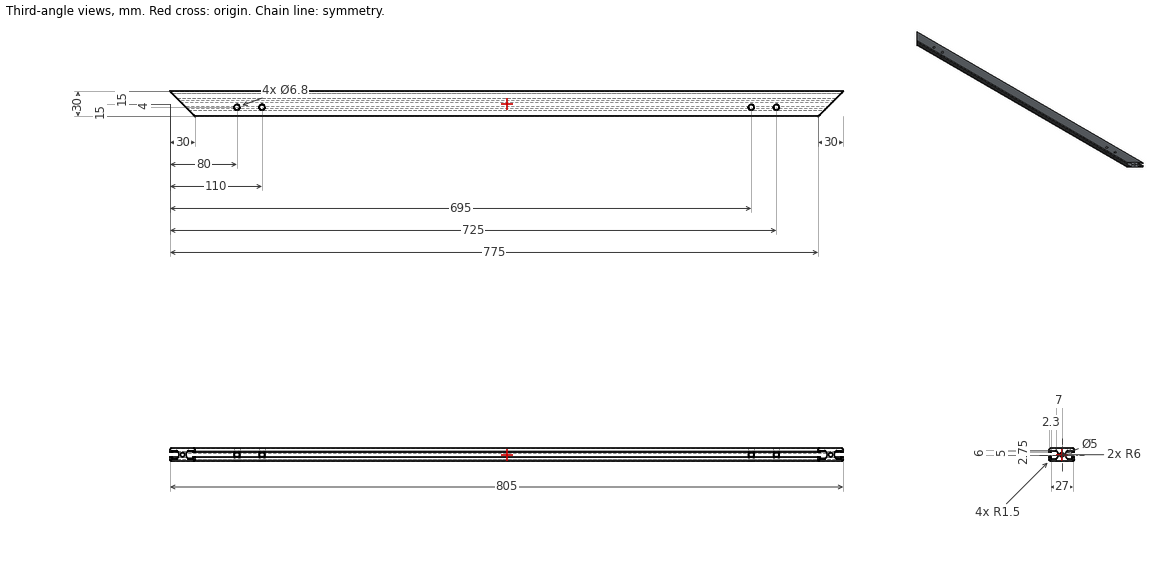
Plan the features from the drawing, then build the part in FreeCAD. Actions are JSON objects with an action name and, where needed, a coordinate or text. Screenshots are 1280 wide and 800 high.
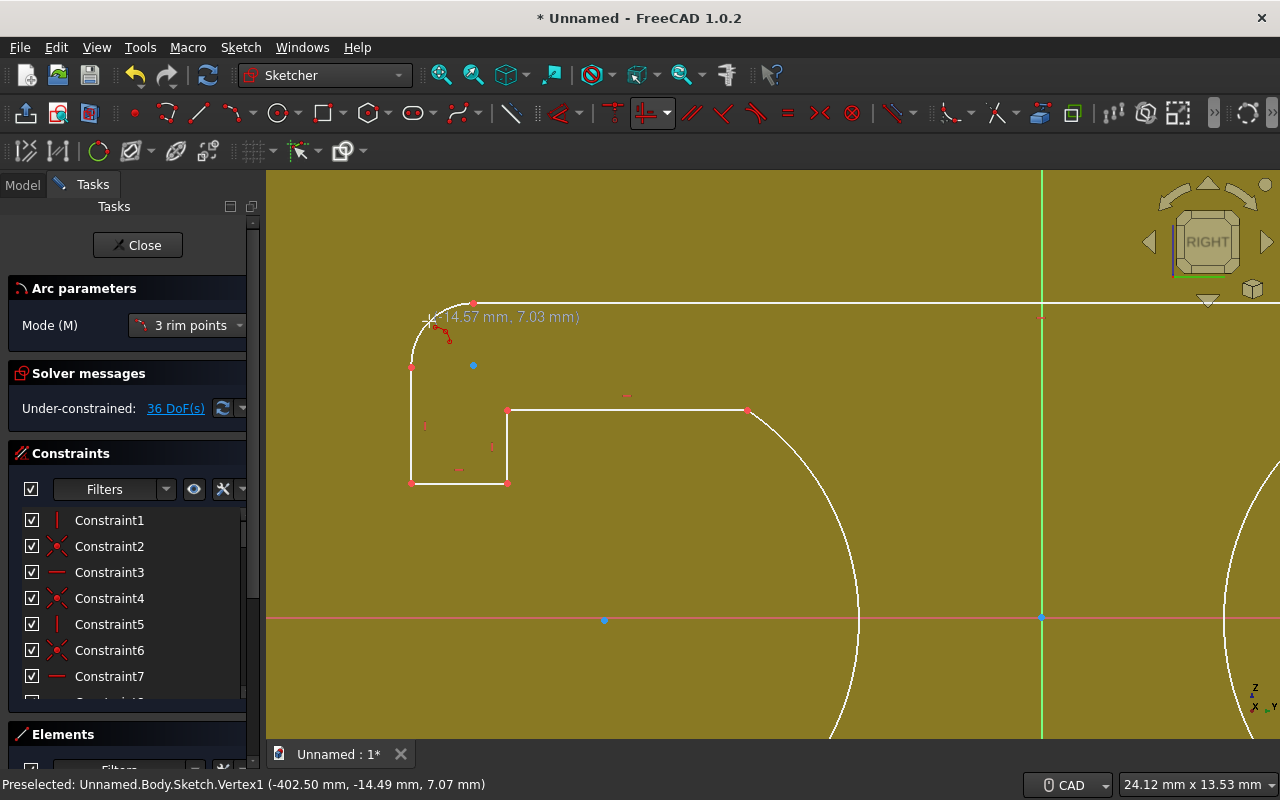
{"action": "left_click", "coordinate": [278, 114]}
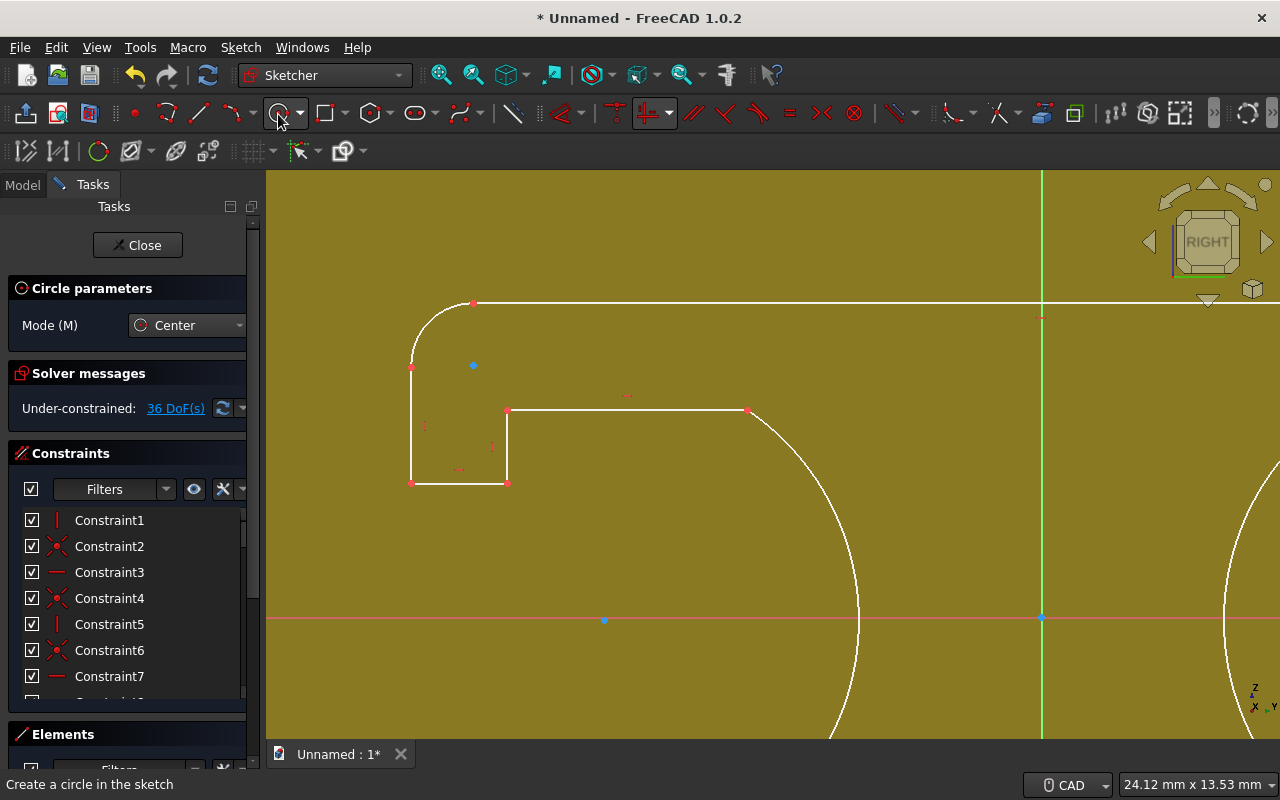
{"action": "left_click", "coordinate": [1042, 618]}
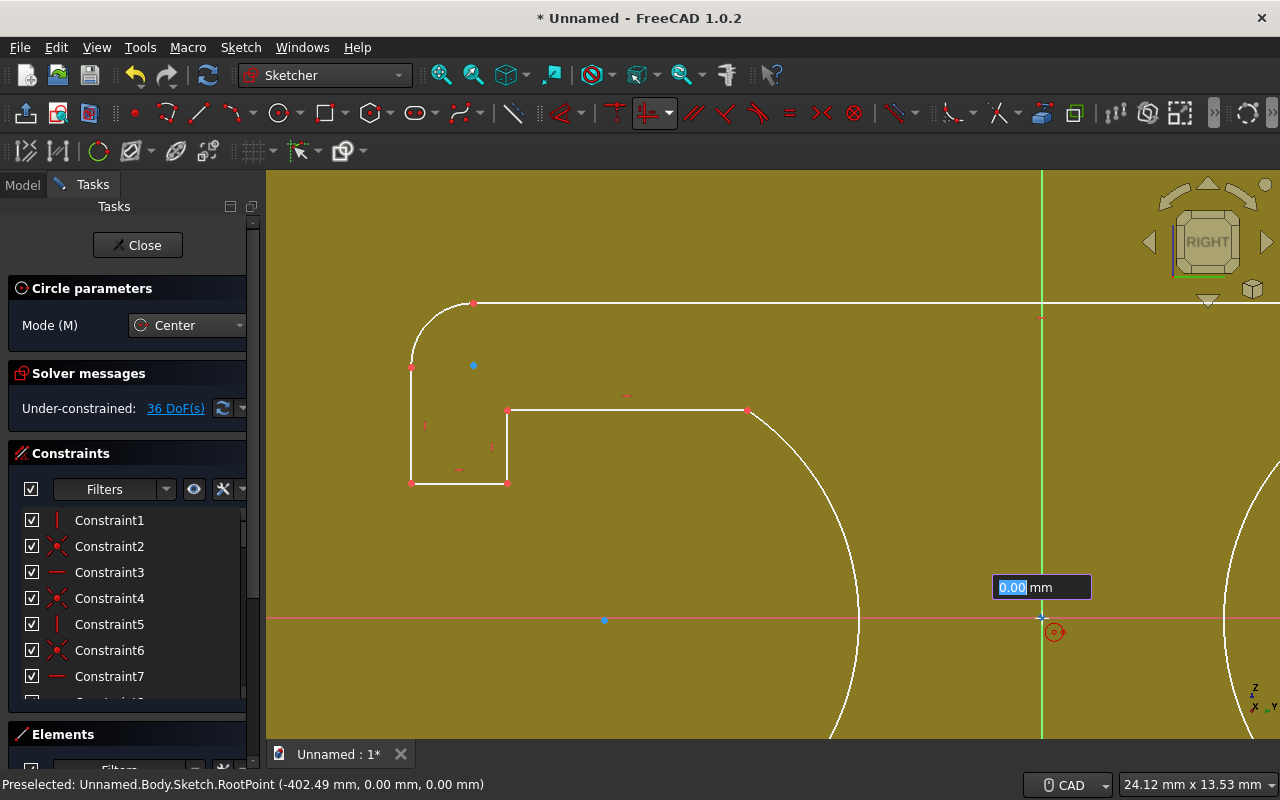
{"action": "scroll", "coordinate": [429, 321], "scroll_direction": "down", "scroll_amount": 4}
{"action": "mouse_move", "coordinate": [738, 421]}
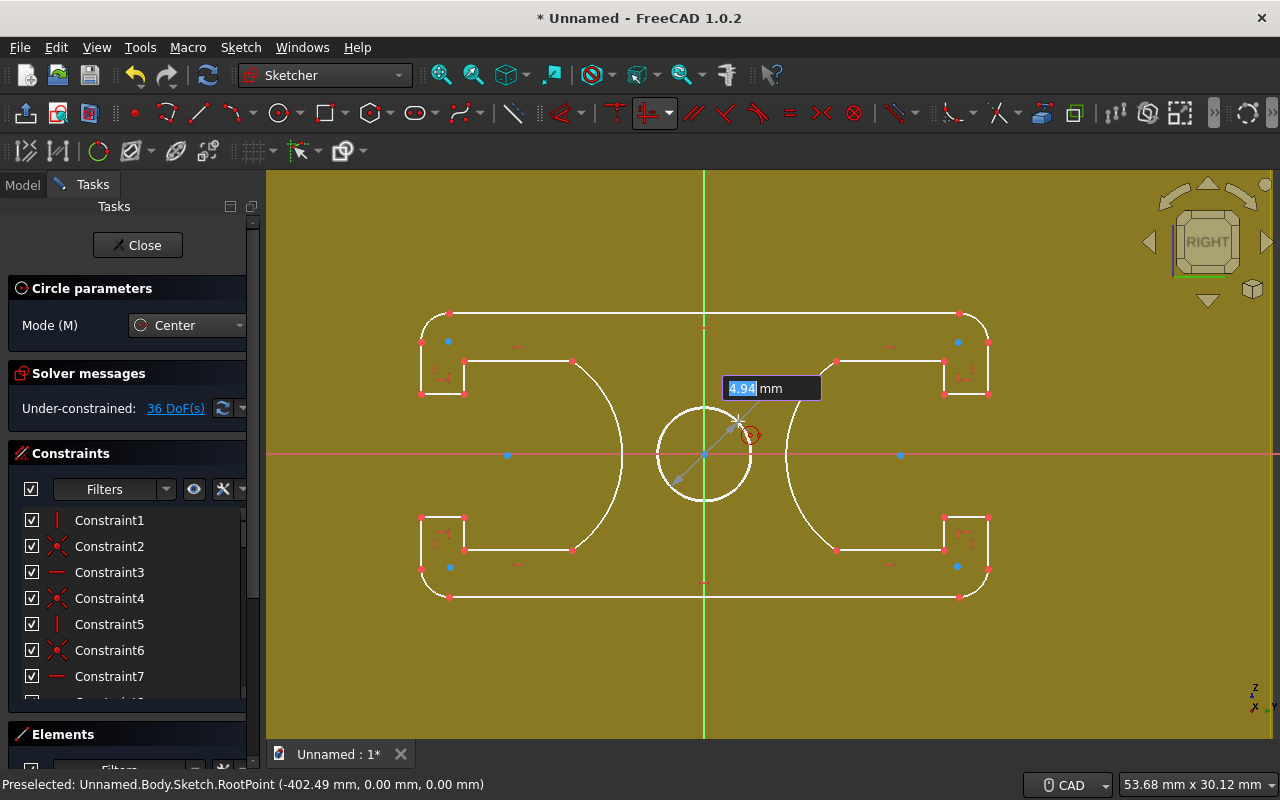
{"action": "type", "text": "5"}
{"action": "key", "text": "Return"}
{"action": "key", "text": "Escape"}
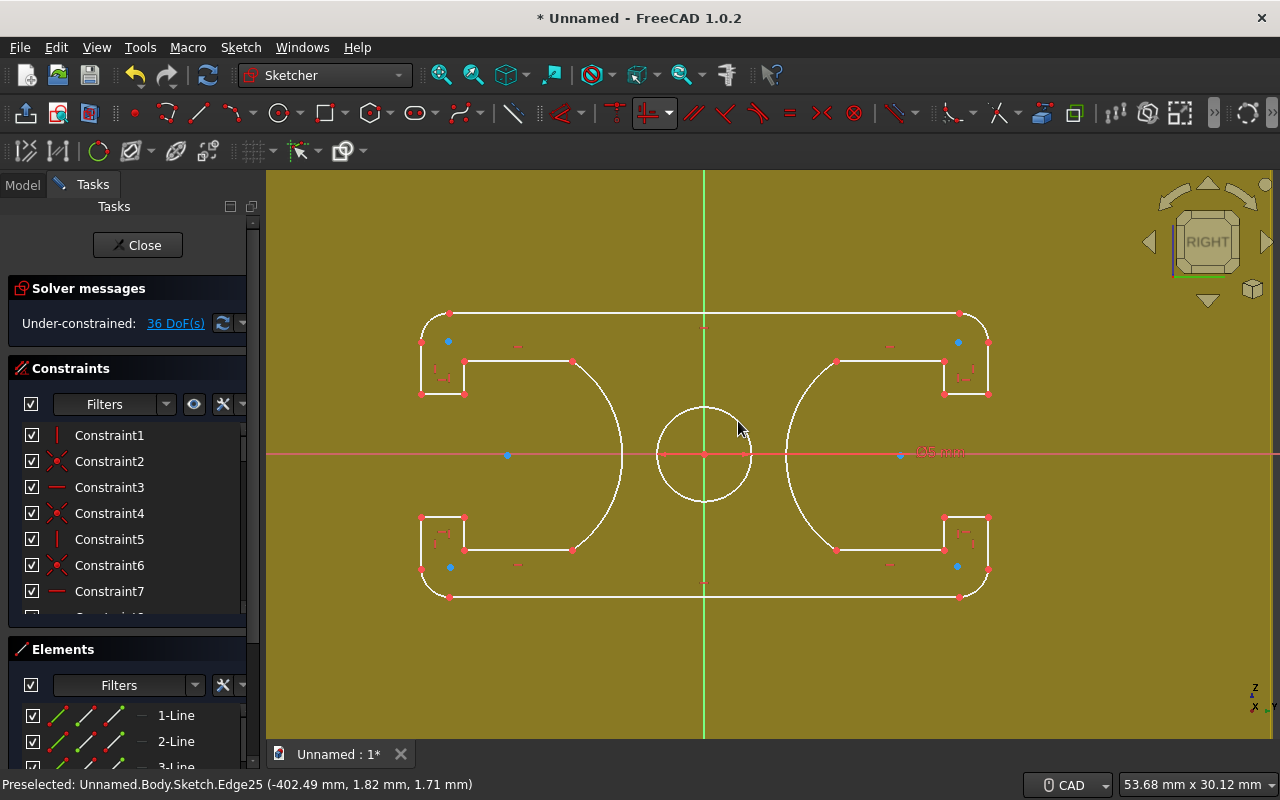
{"action": "left_click", "coordinate": [421, 358]}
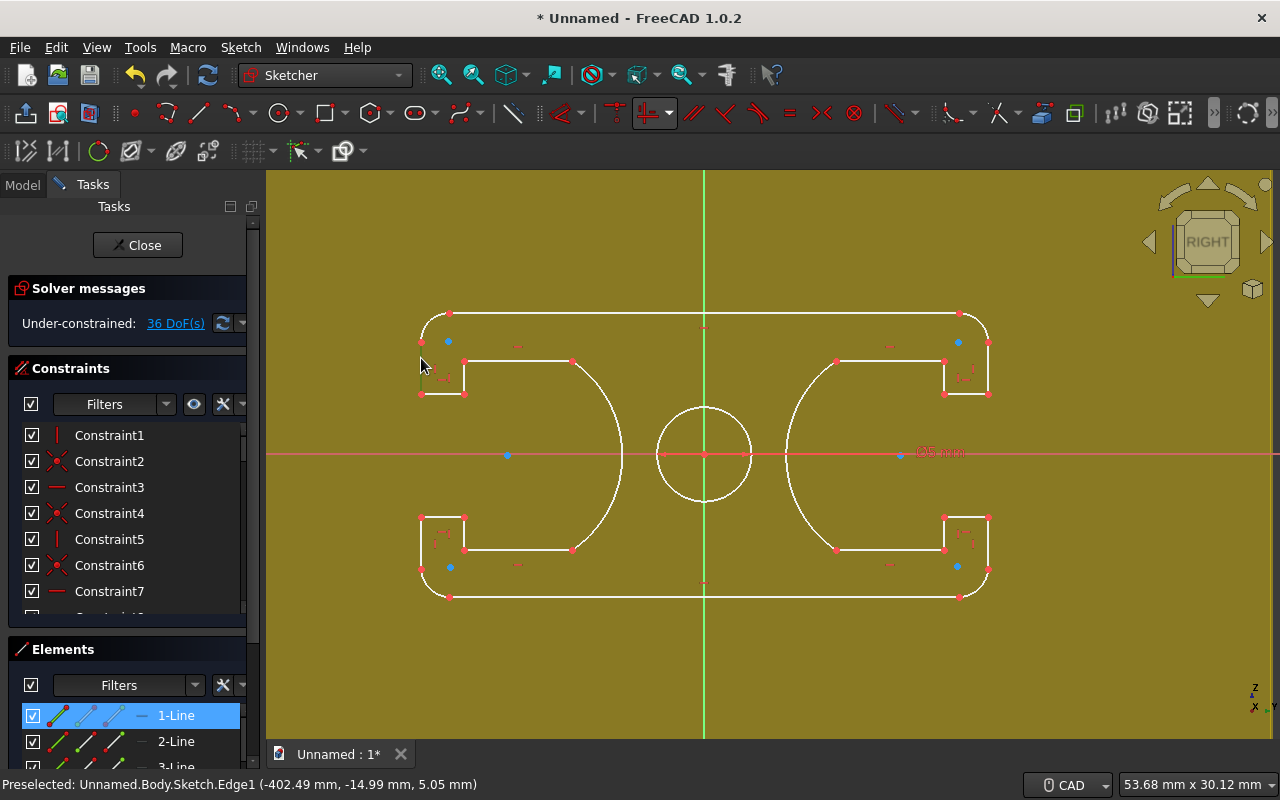
{"action": "left_click", "coordinate": [436, 316]}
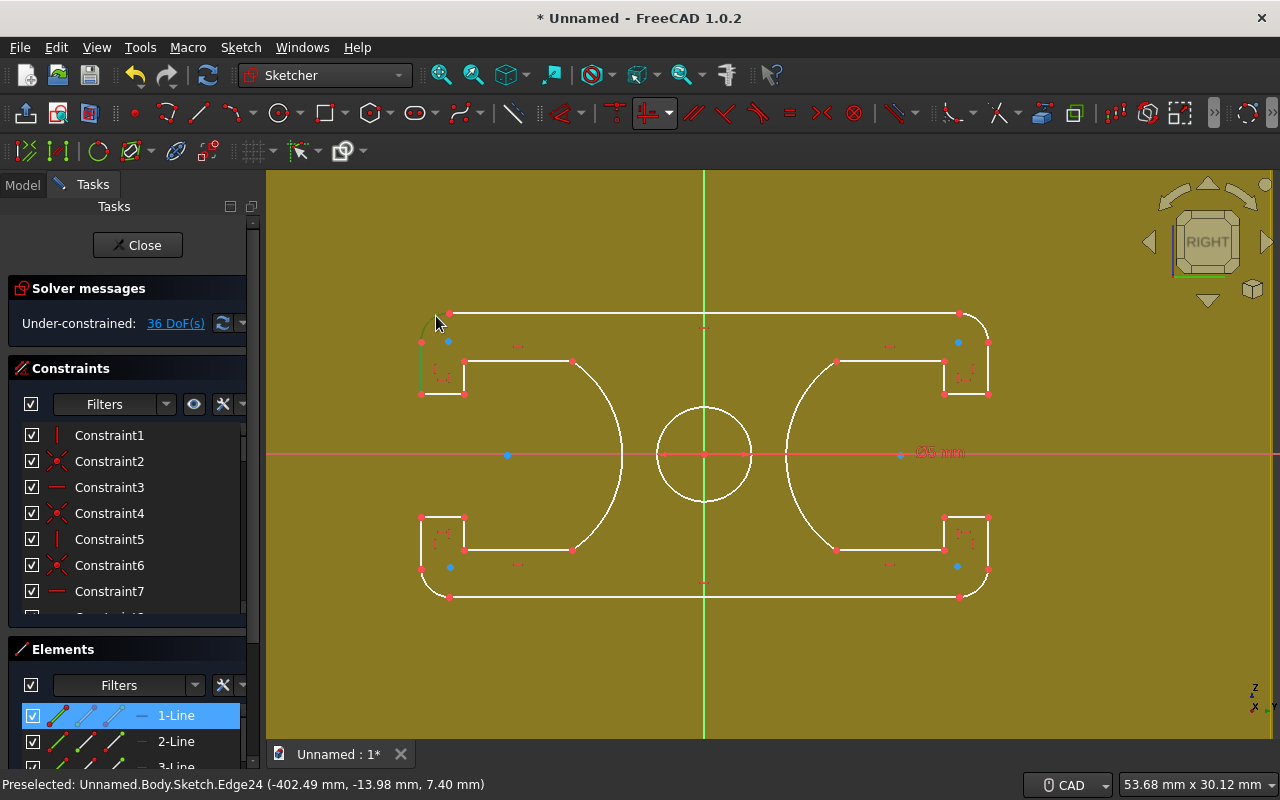
{"action": "left_click", "coordinate": [758, 114]}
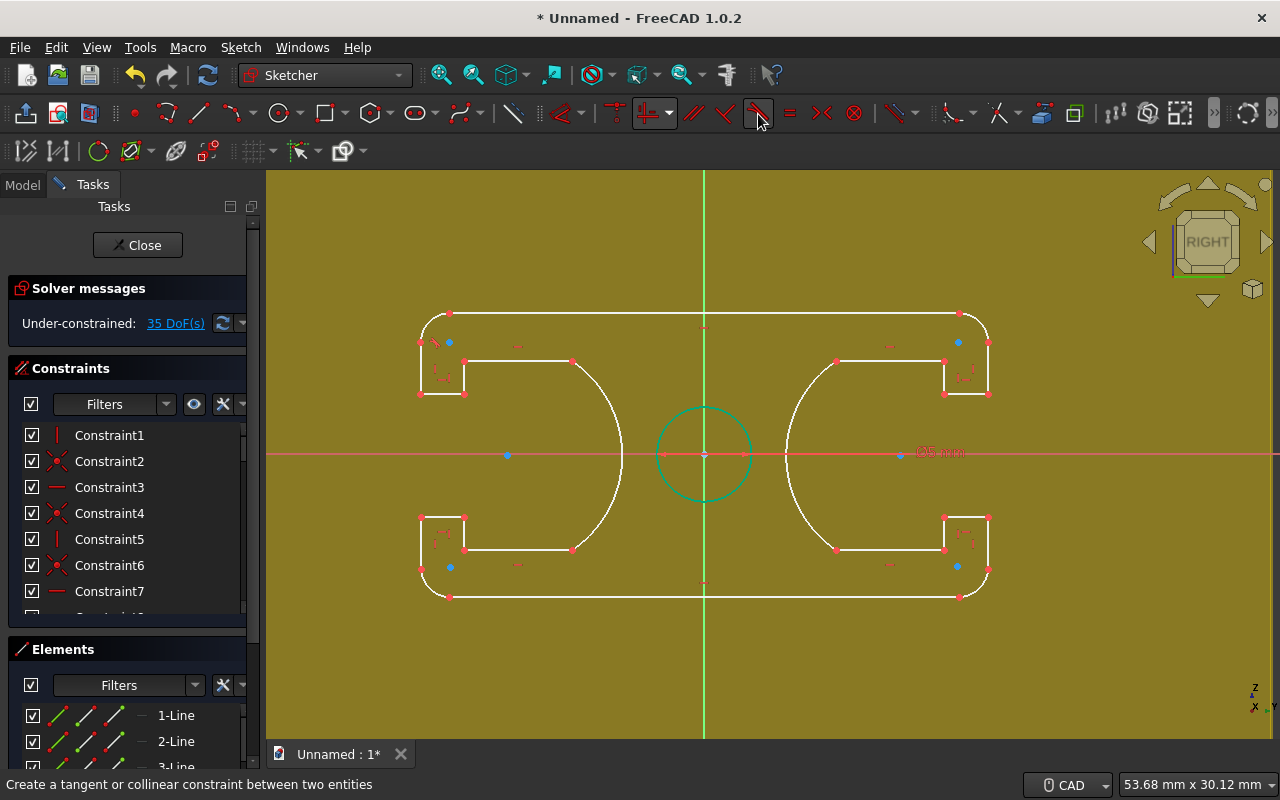
{"action": "left_click", "coordinate": [421, 533]}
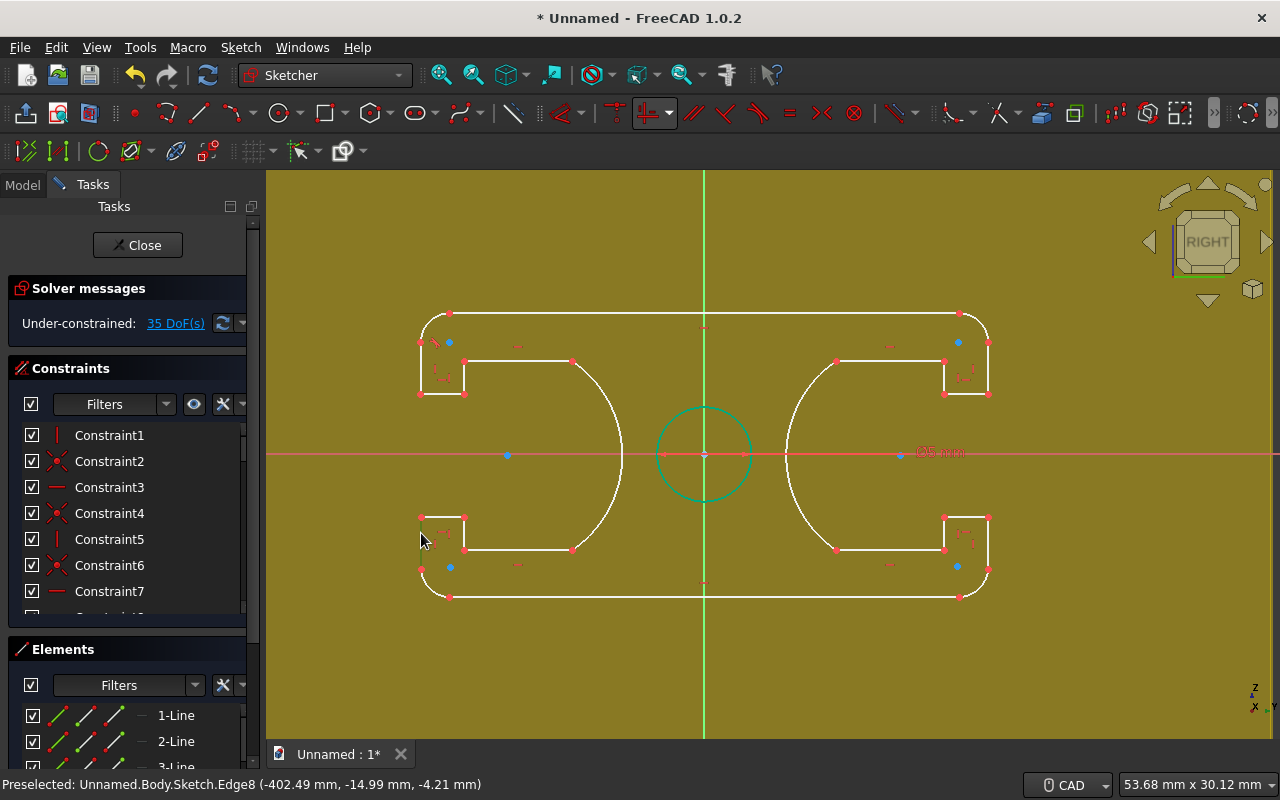
{"action": "left_click", "coordinate": [425, 582]}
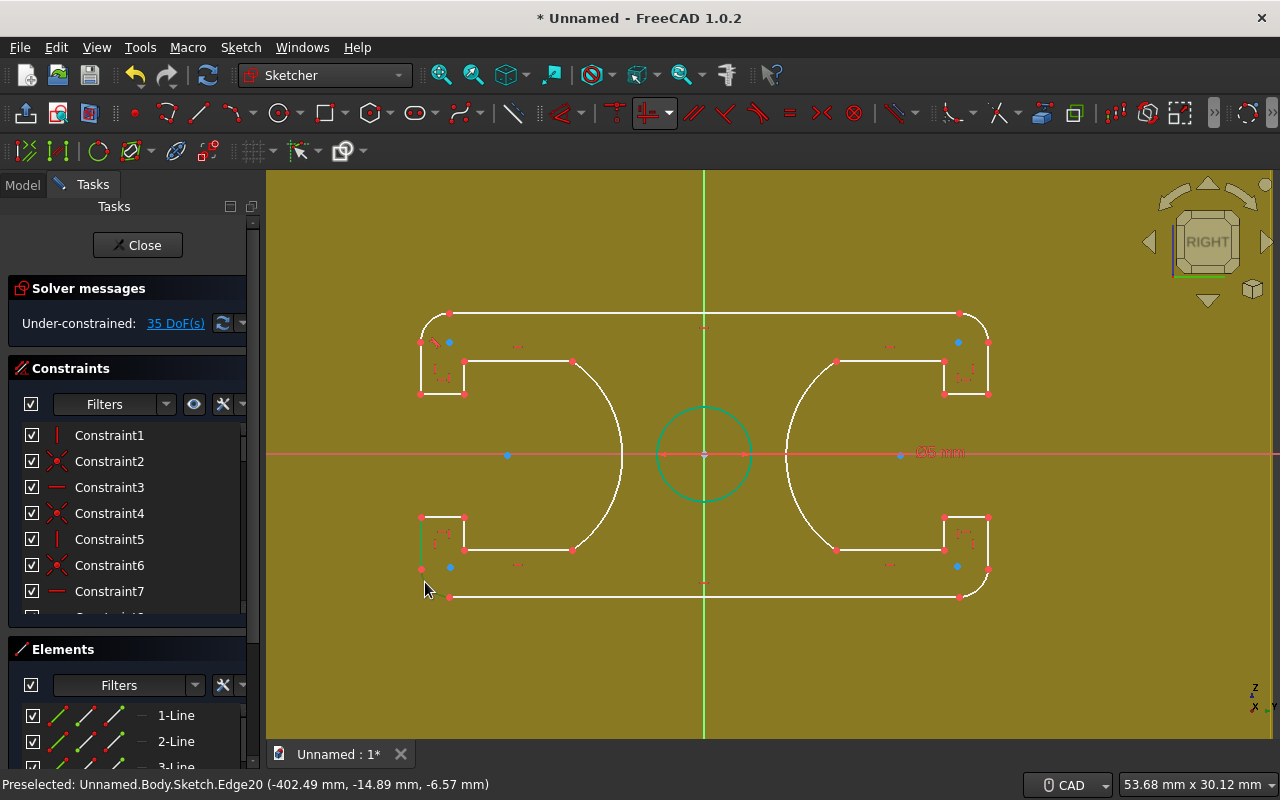
{"action": "left_click", "coordinate": [758, 114]}